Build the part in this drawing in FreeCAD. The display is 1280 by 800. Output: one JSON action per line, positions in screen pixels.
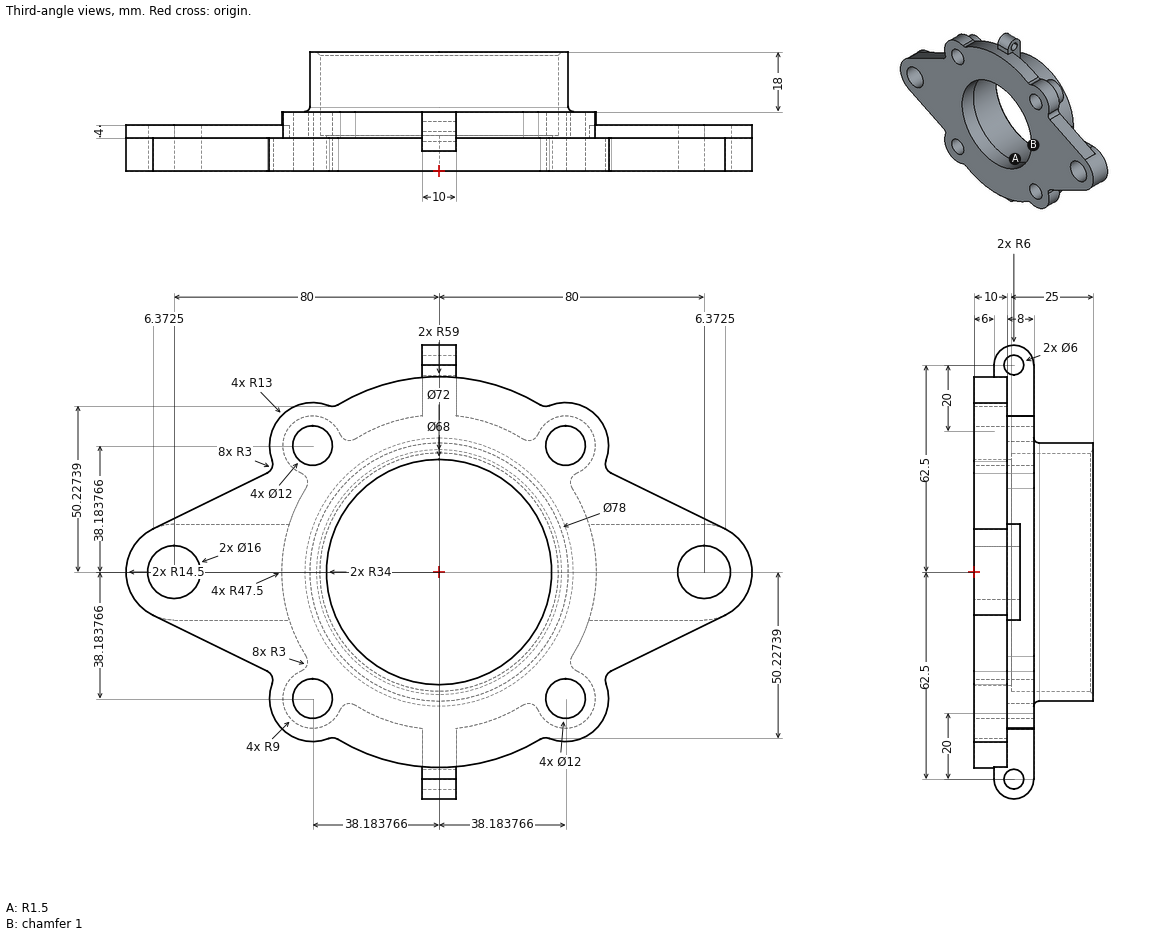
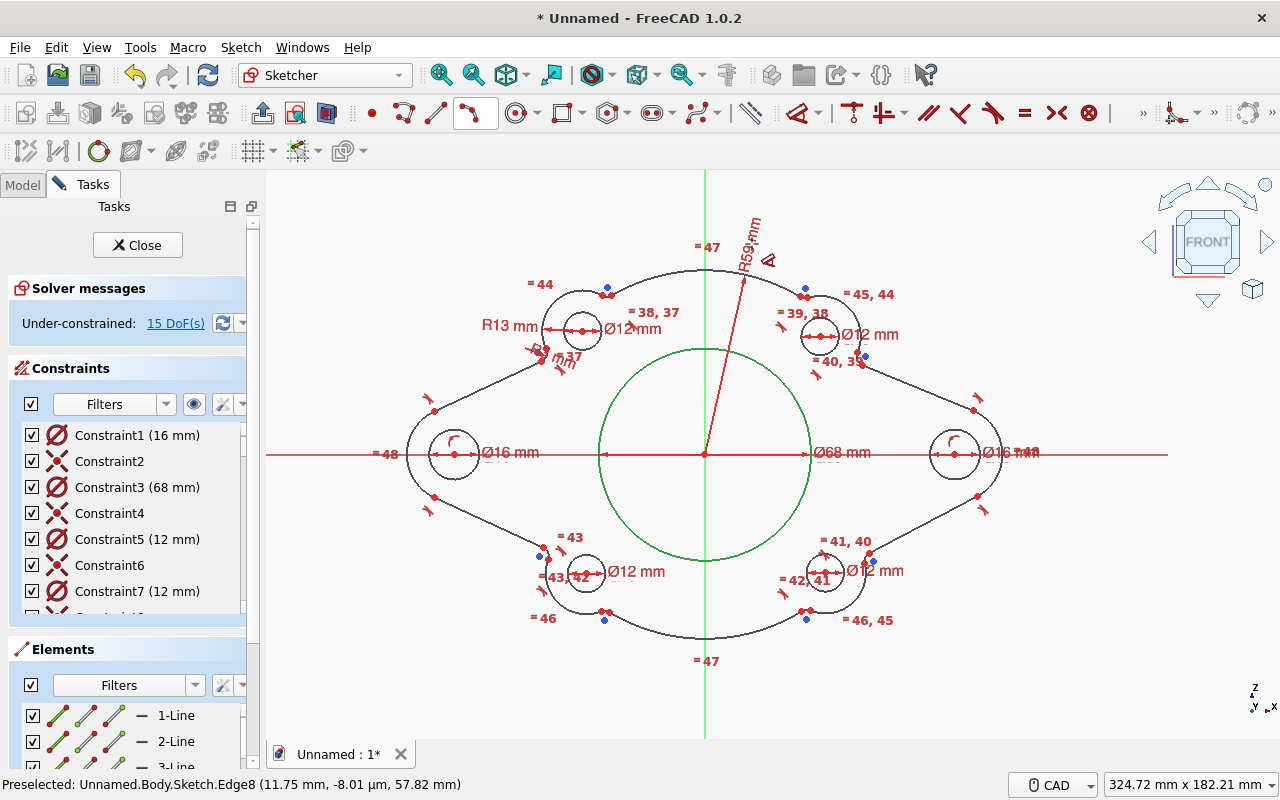
{"action": "left_click", "coordinate": [998, 473]}
{"action": "left_click", "coordinate": [1027, 486]}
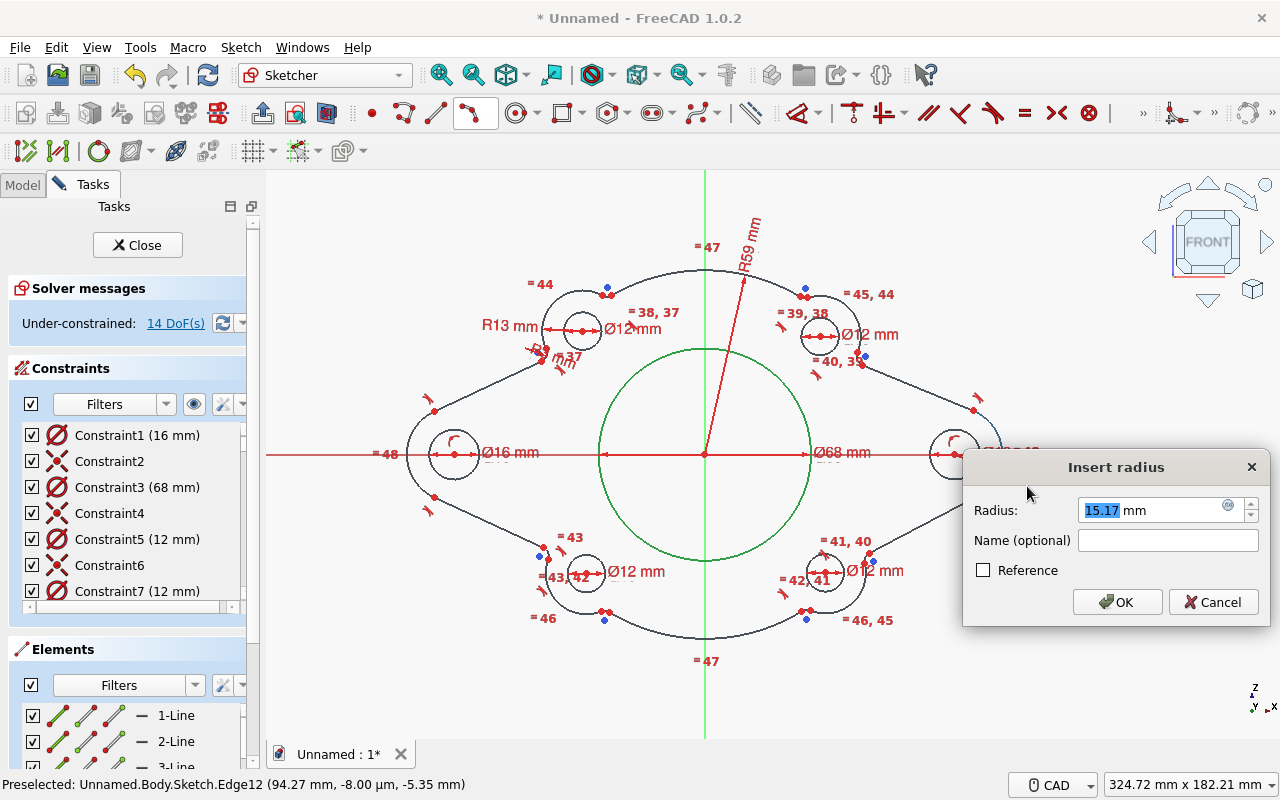
{"action": "type", "text": "14.5"}
{"action": "key", "text": "Return"}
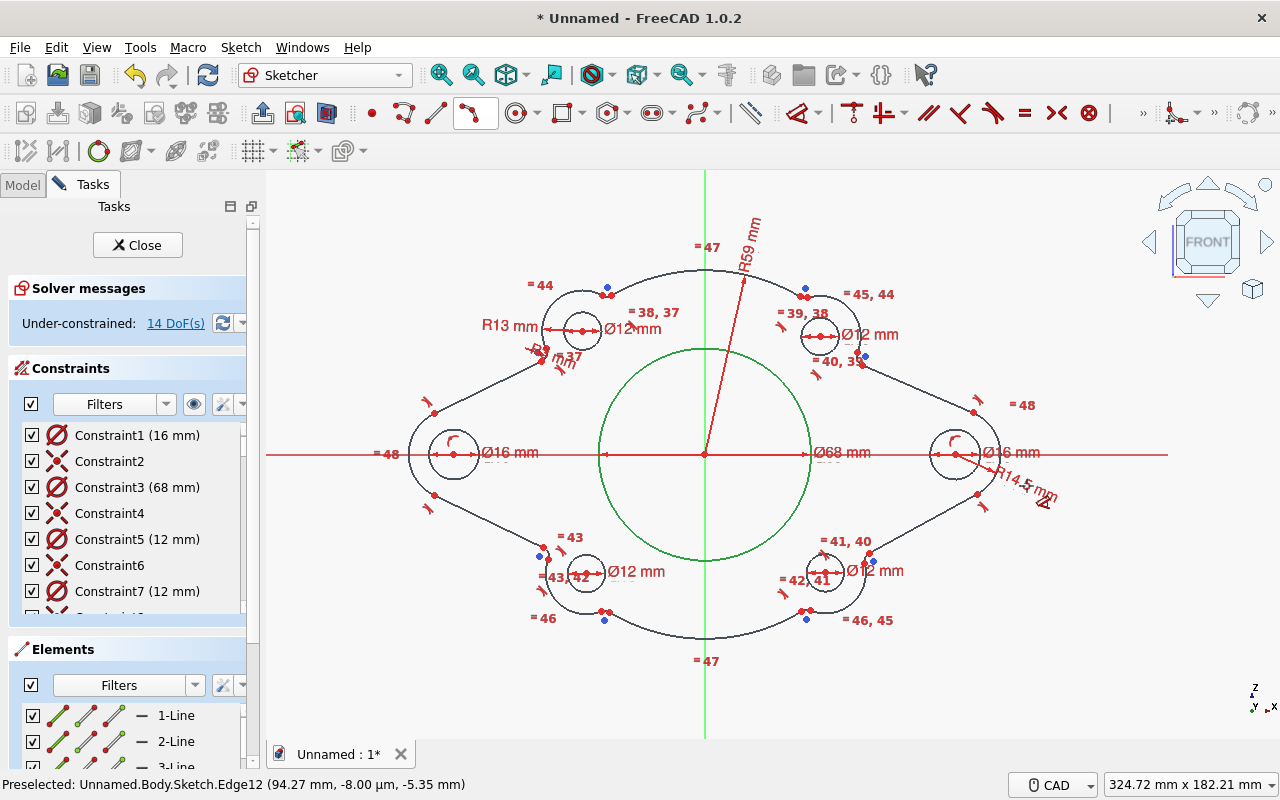
{"action": "left_click", "coordinate": [454, 455]}
{"action": "left_click", "coordinate": [579, 489]}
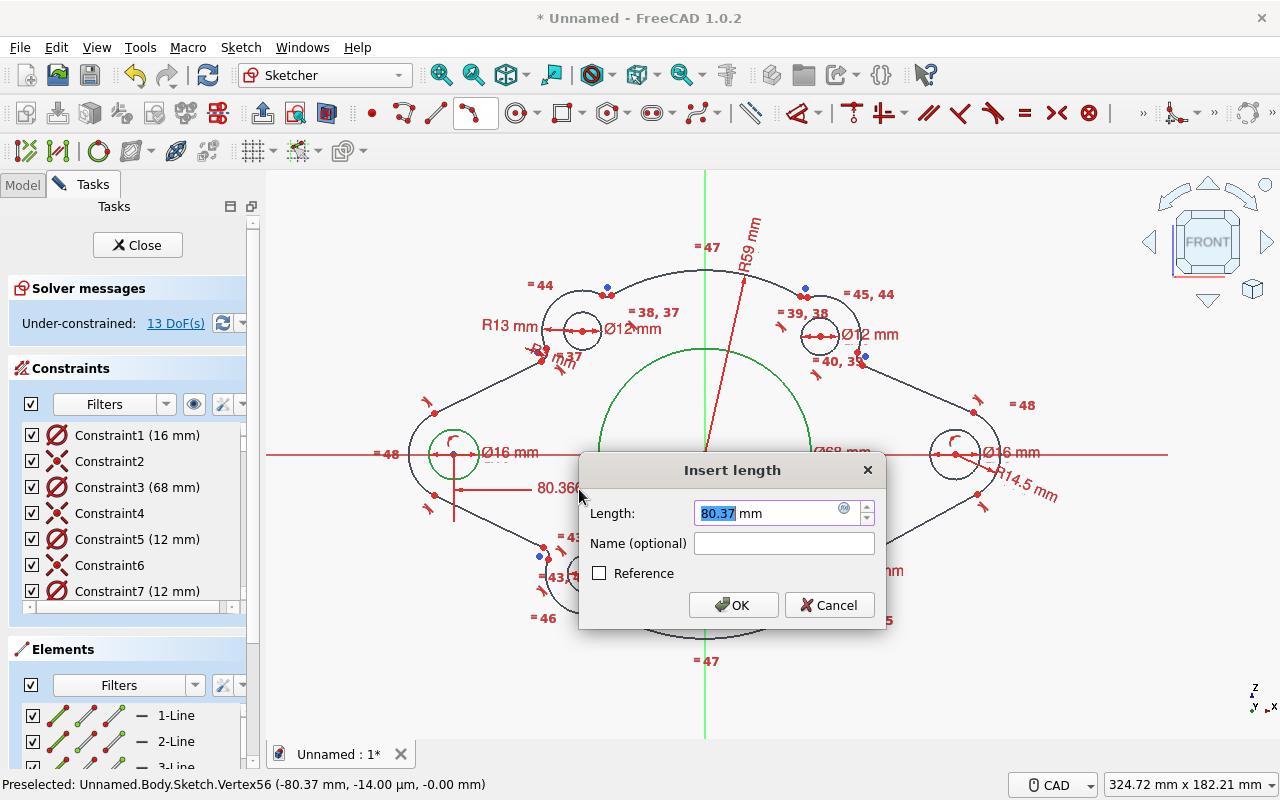
{"action": "type", "text": "80"}
{"action": "key", "text": "Return"}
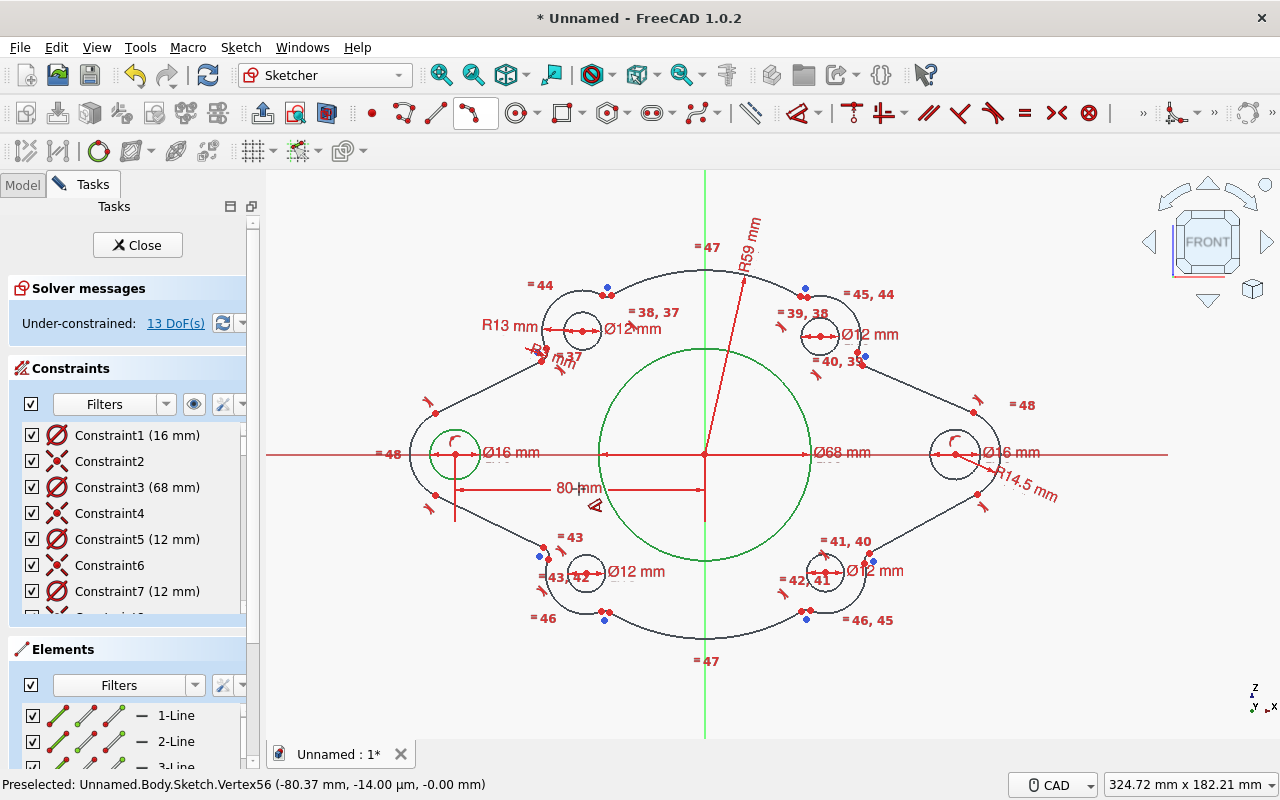
{"action": "left_click", "coordinate": [955, 455]}
{"action": "left_click", "coordinate": [830, 489]}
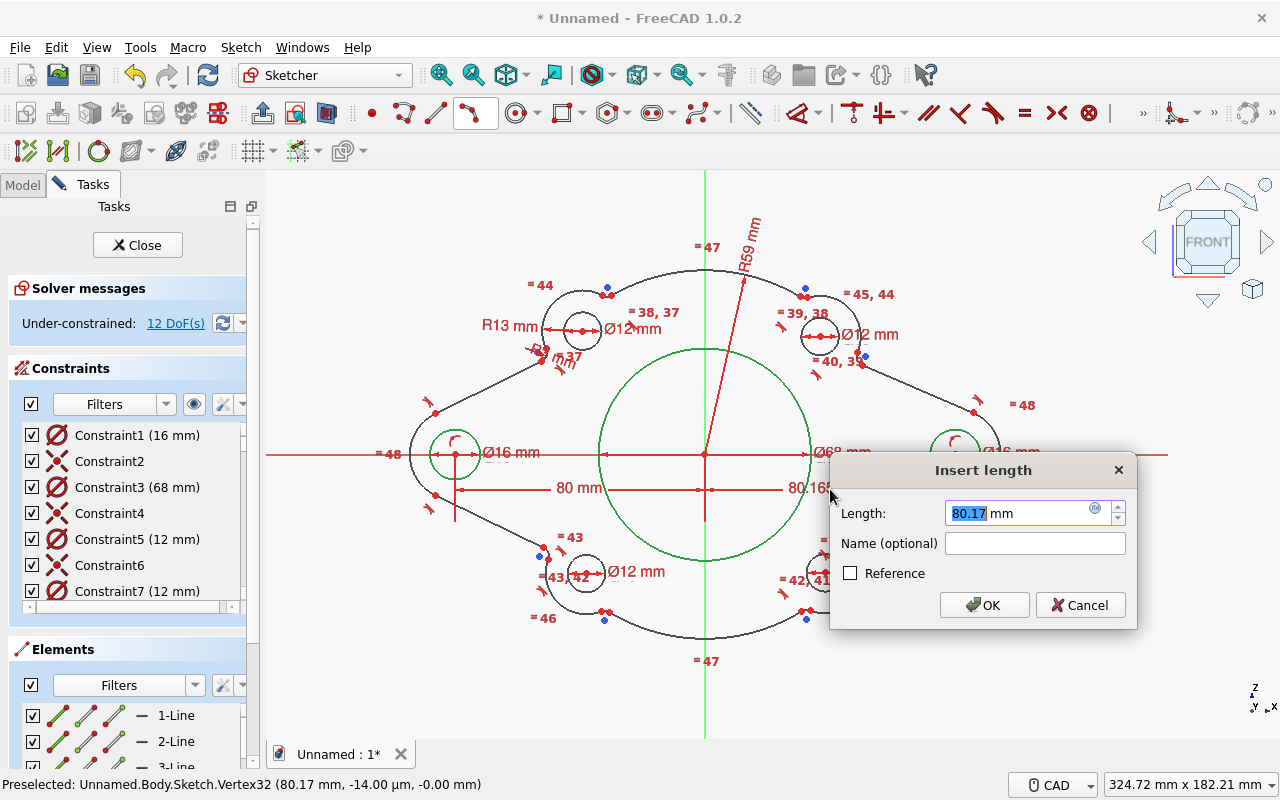
{"action": "type", "text": "80"}
{"action": "key", "text": "Return"}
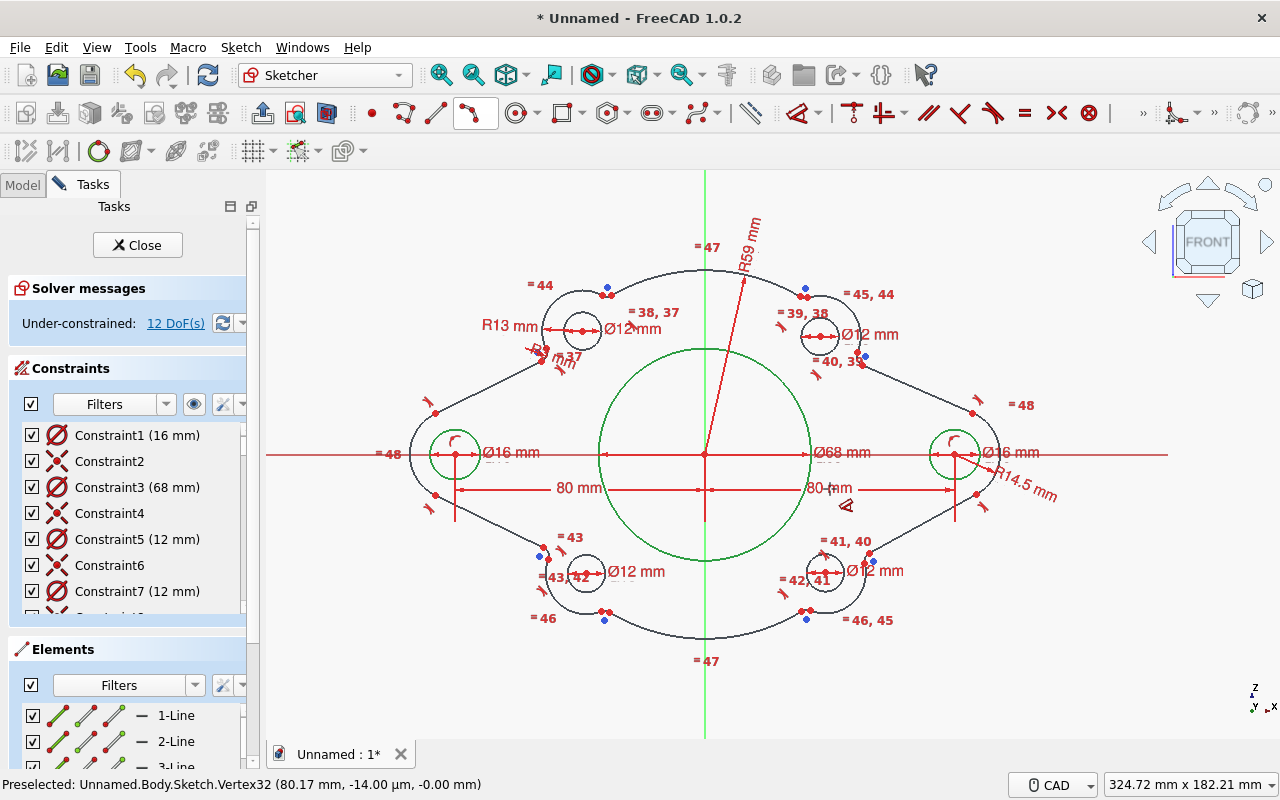
{"action": "scroll", "coordinate": [435, 414], "scroll_direction": "up", "scroll_amount": 4}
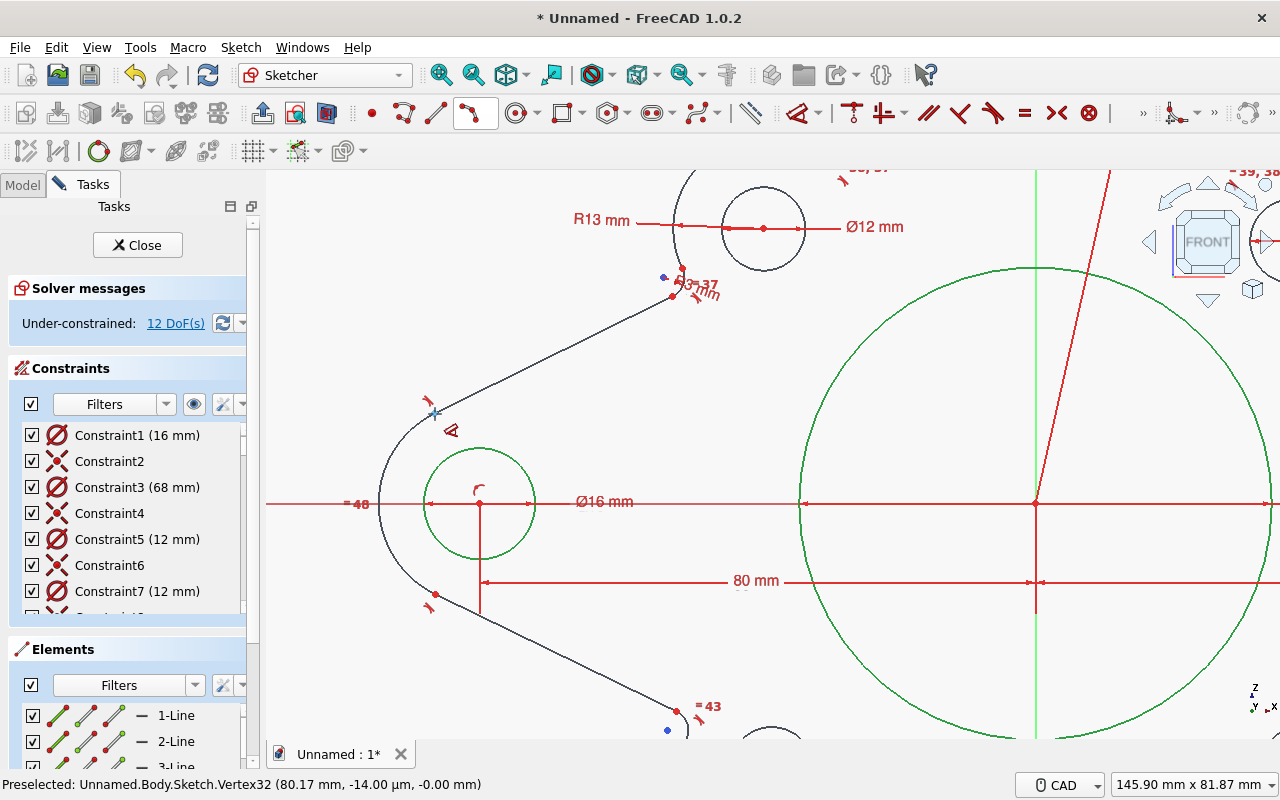
{"action": "left_click", "coordinate": [435, 413]}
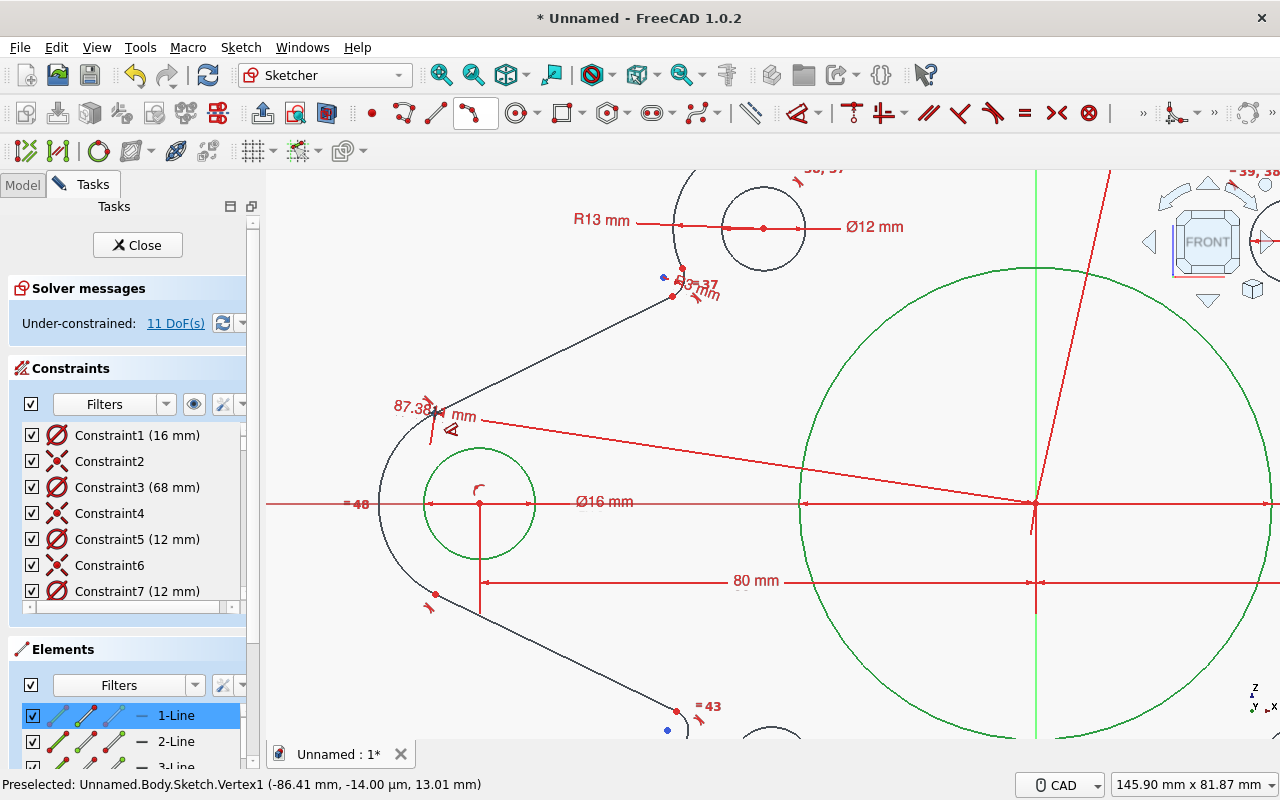
{"action": "left_click", "coordinate": [480, 504]}
{"action": "left_click", "coordinate": [457, 379]}